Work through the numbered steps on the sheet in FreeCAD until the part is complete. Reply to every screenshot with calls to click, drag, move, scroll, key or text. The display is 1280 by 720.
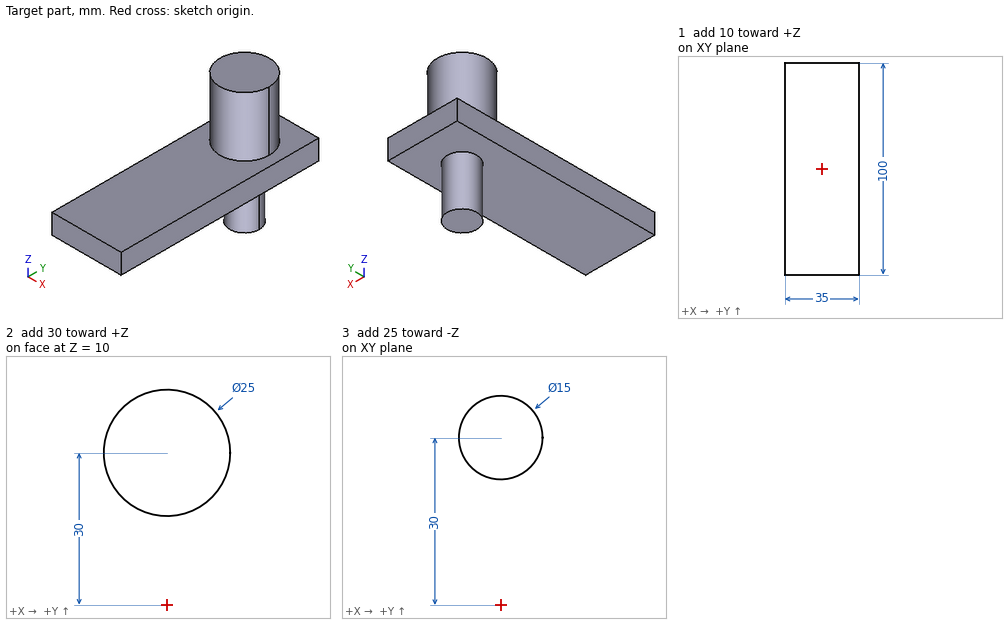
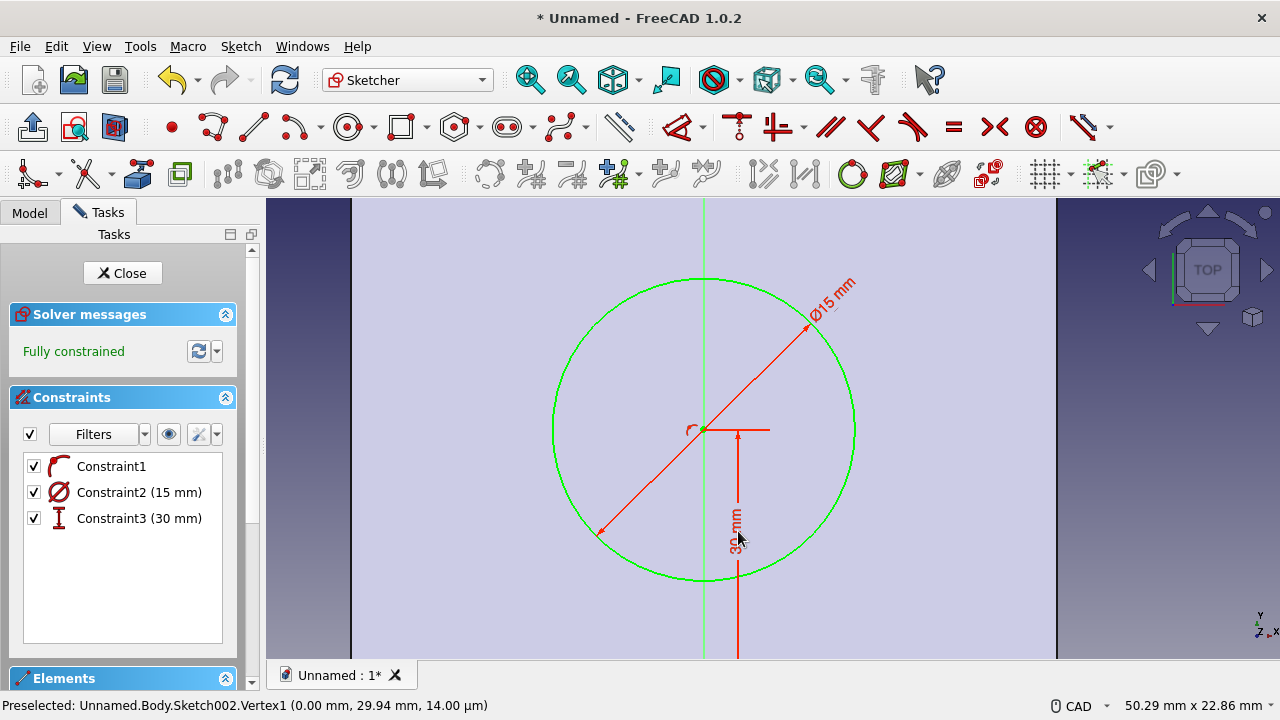
click(123, 273)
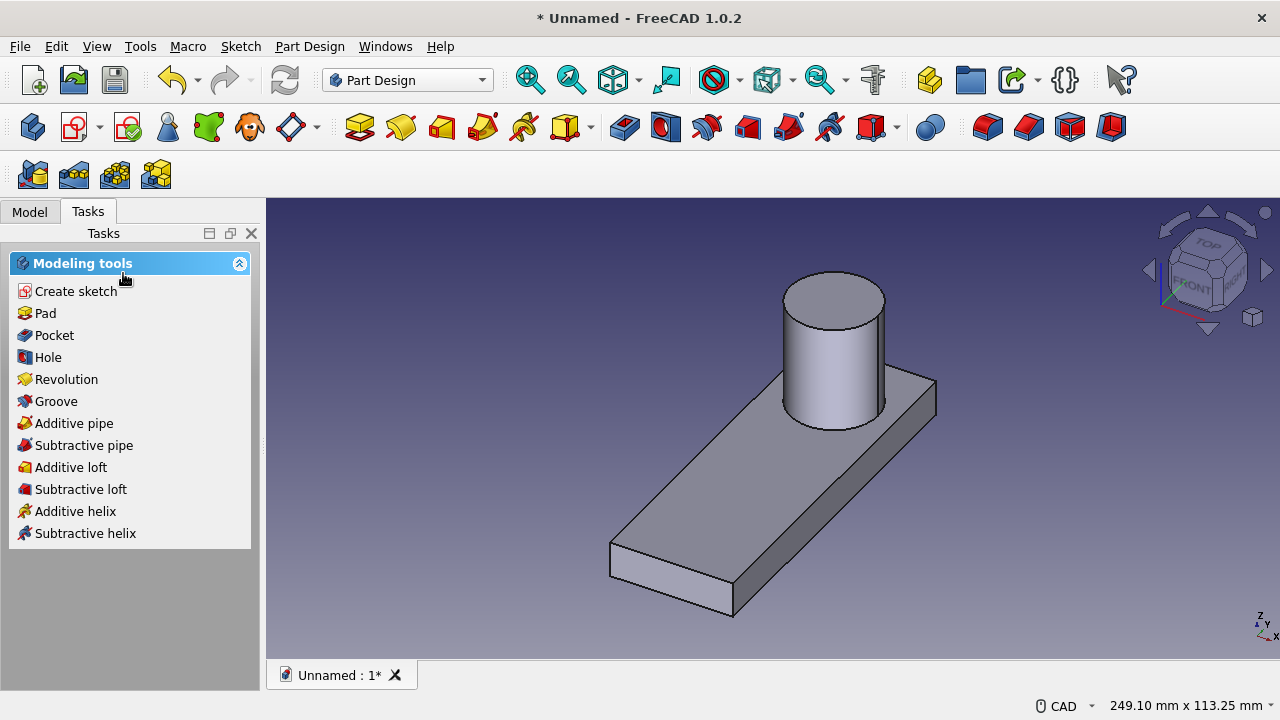
click(360, 128)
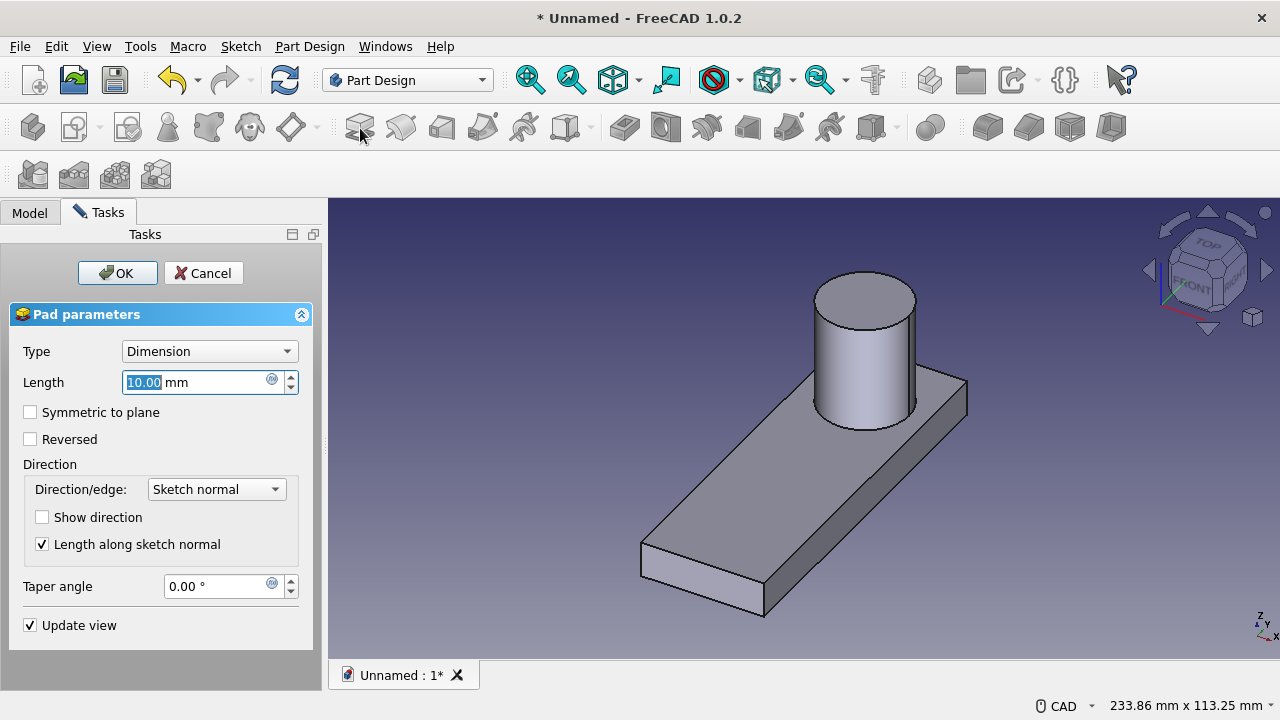
text(25)
key(Tab)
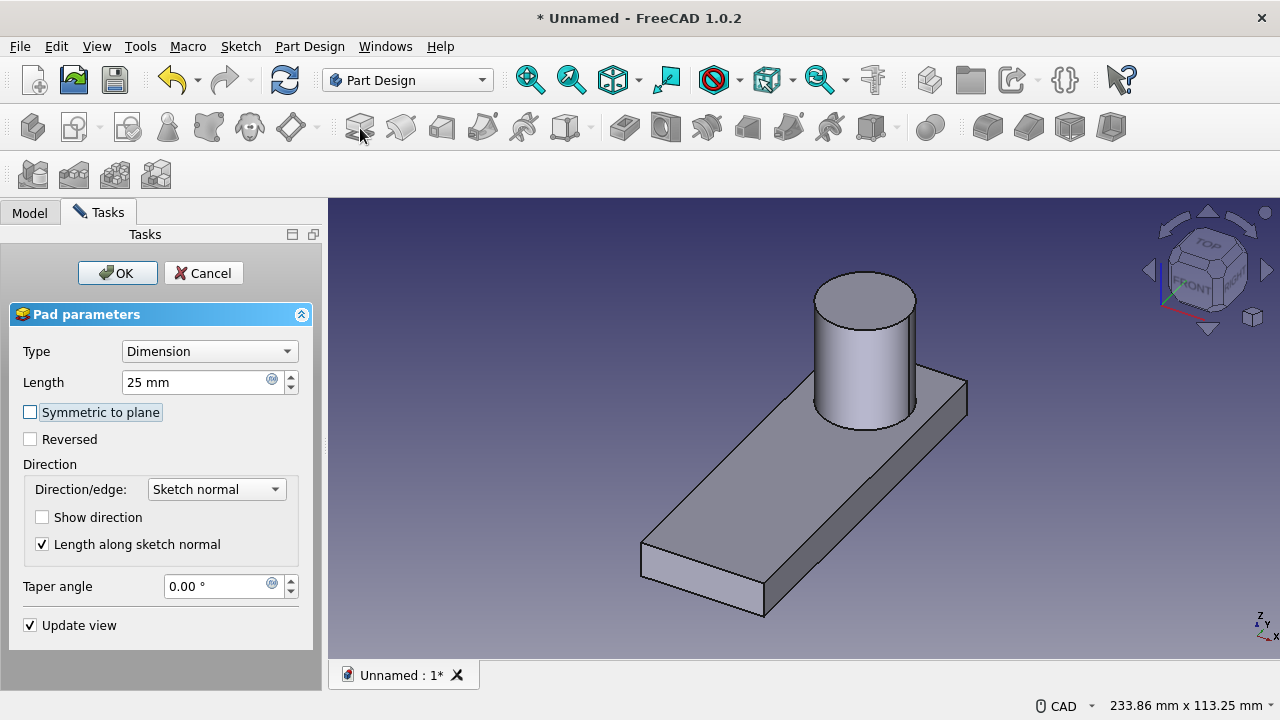
click(31, 439)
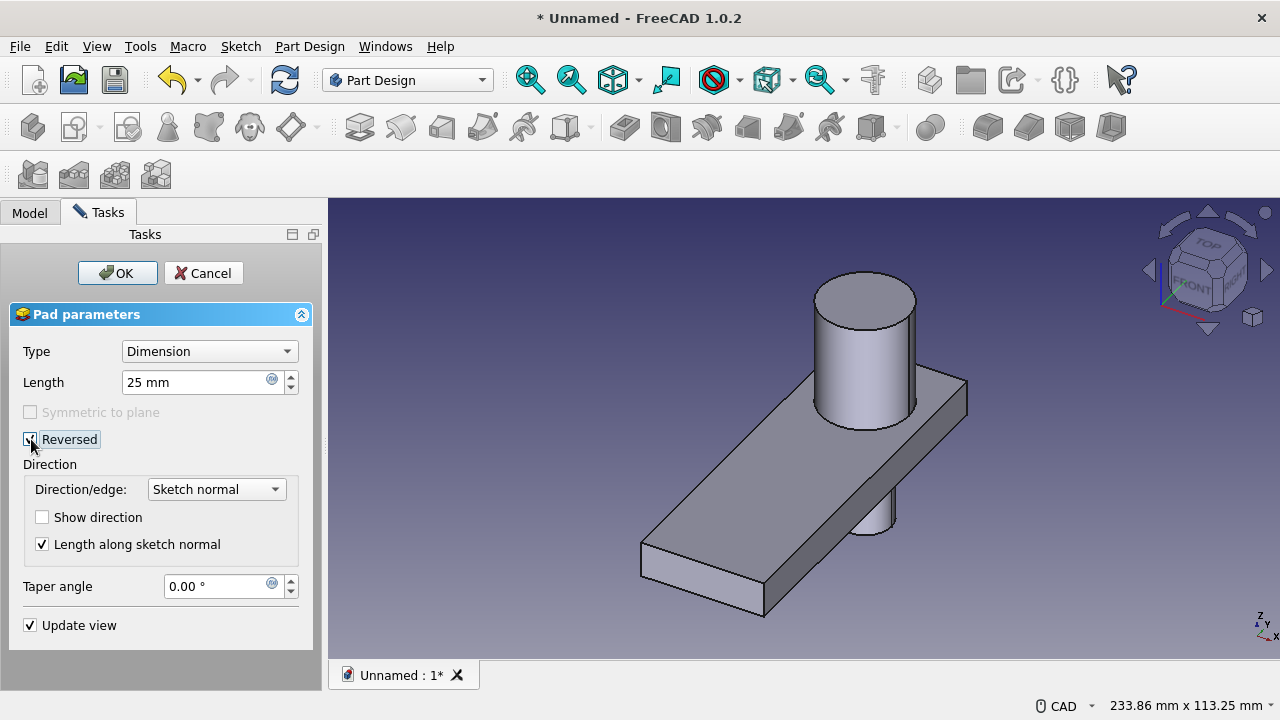
click(118, 273)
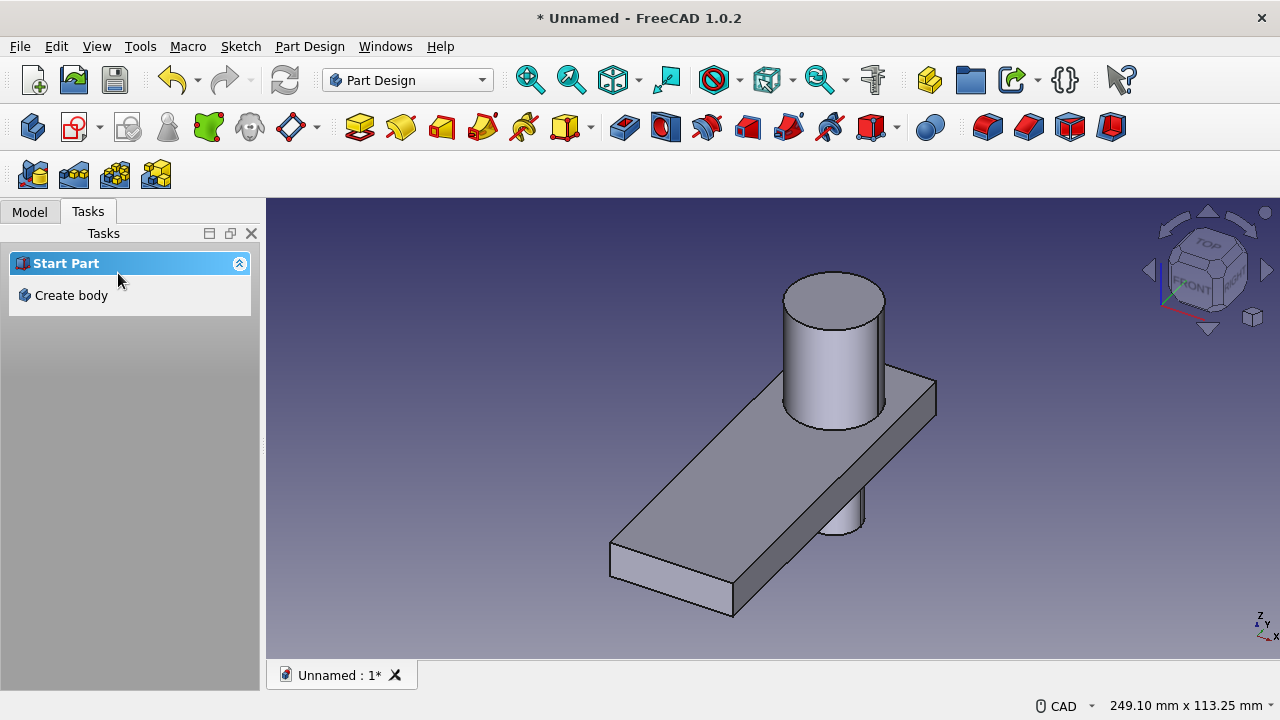
key(0)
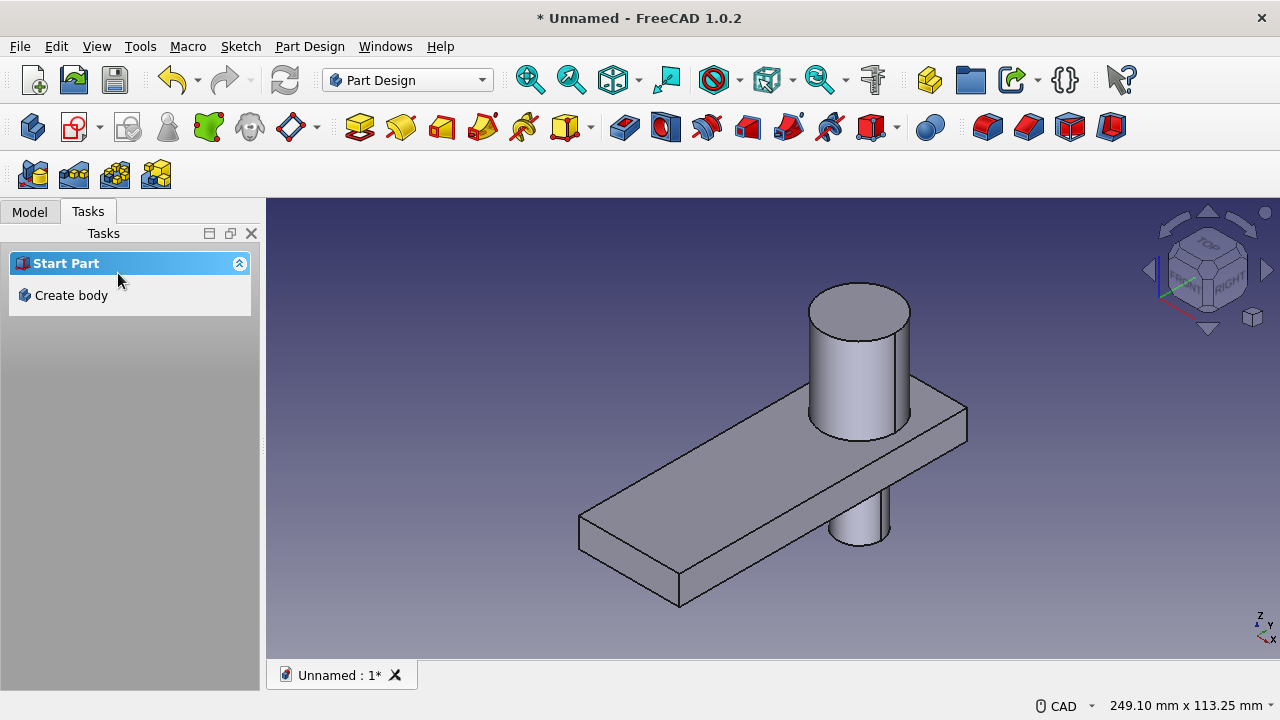
key(v)
key(f)